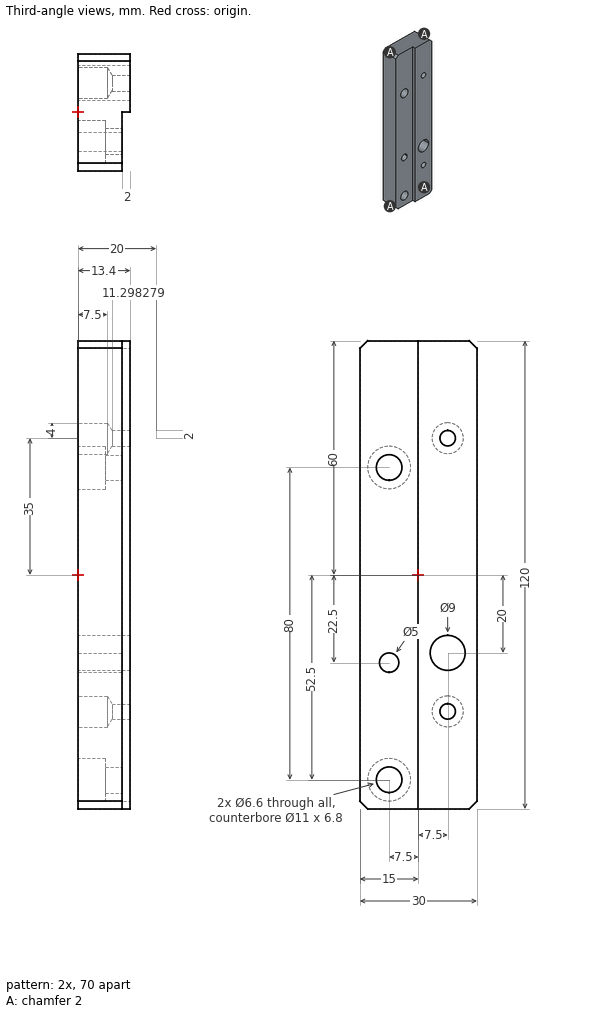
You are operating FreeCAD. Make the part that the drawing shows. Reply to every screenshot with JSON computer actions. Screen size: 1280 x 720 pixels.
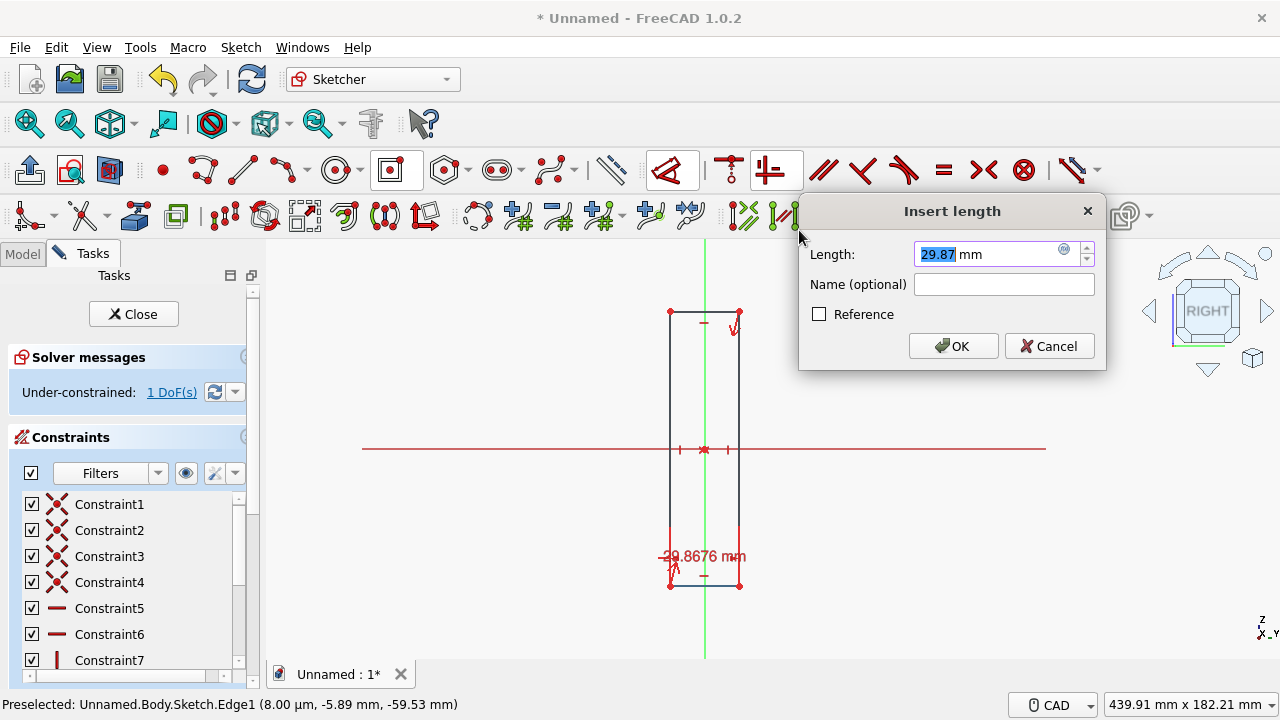
{"action": "type", "text": "30"}
{"action": "key", "text": "Return"}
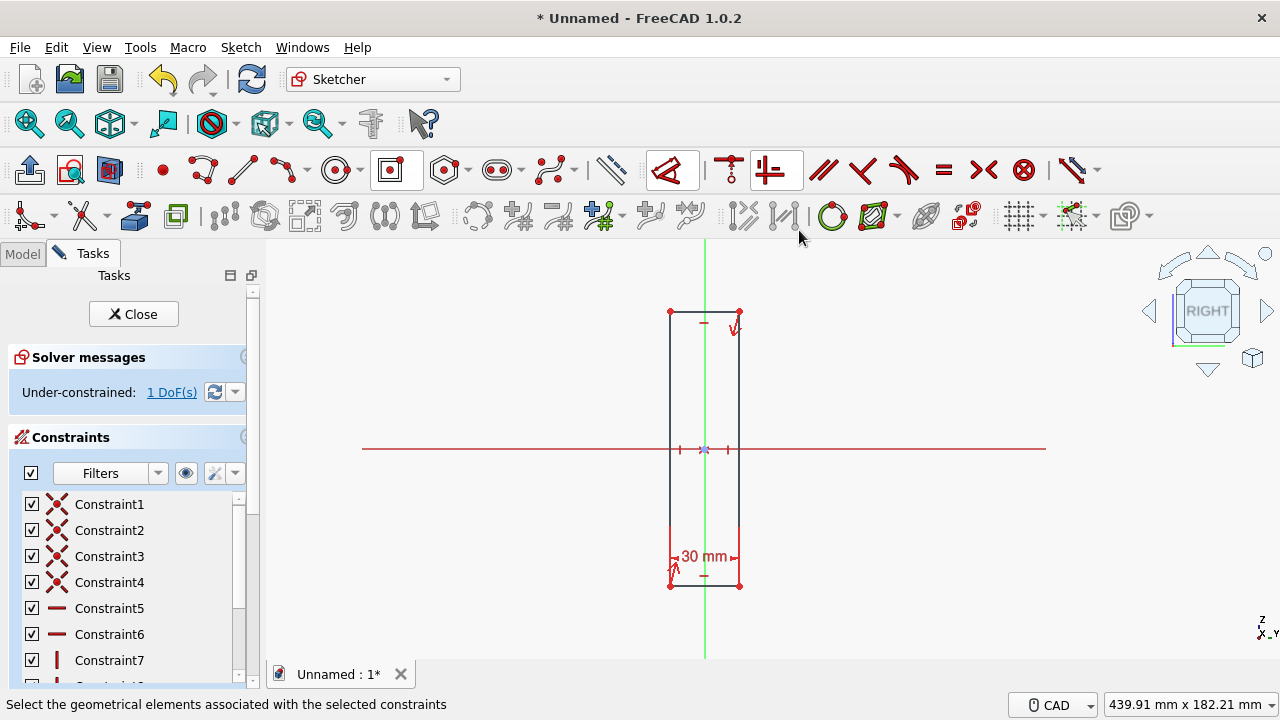
{"action": "left_click", "coordinate": [739, 504]}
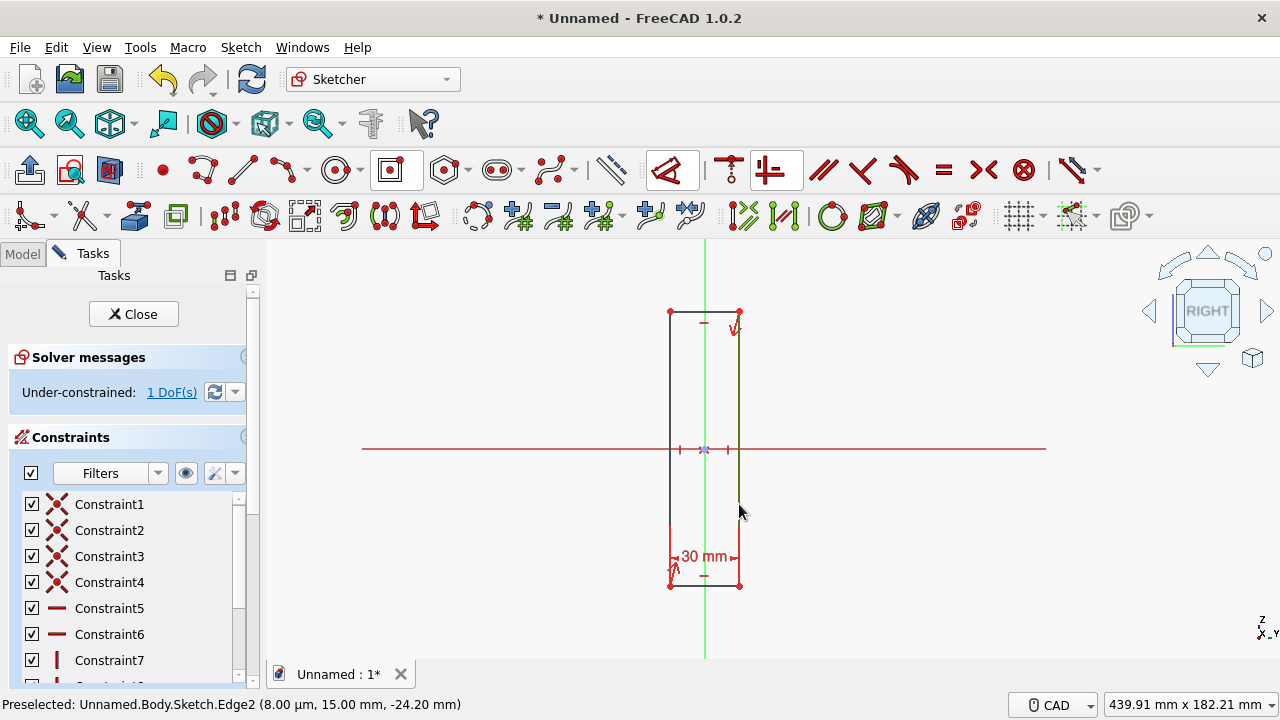
{"action": "key", "text": "i"}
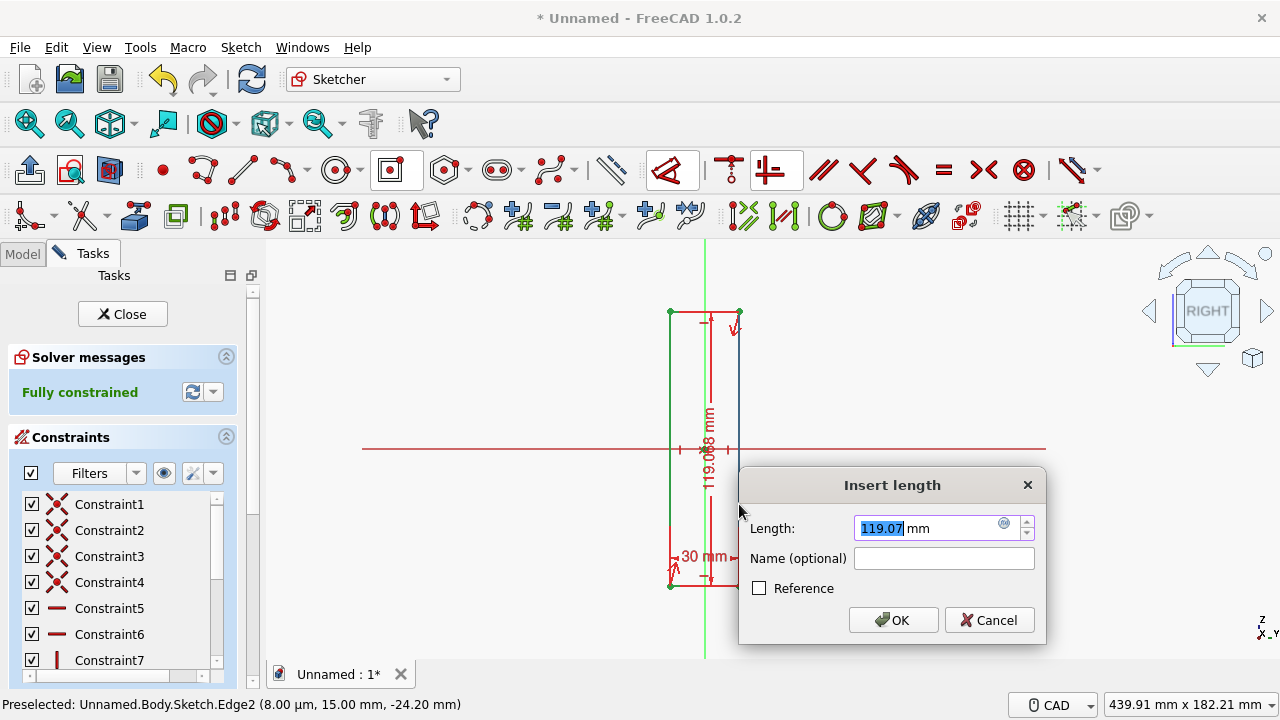
{"action": "type", "text": "120"}
{"action": "key", "text": "Return"}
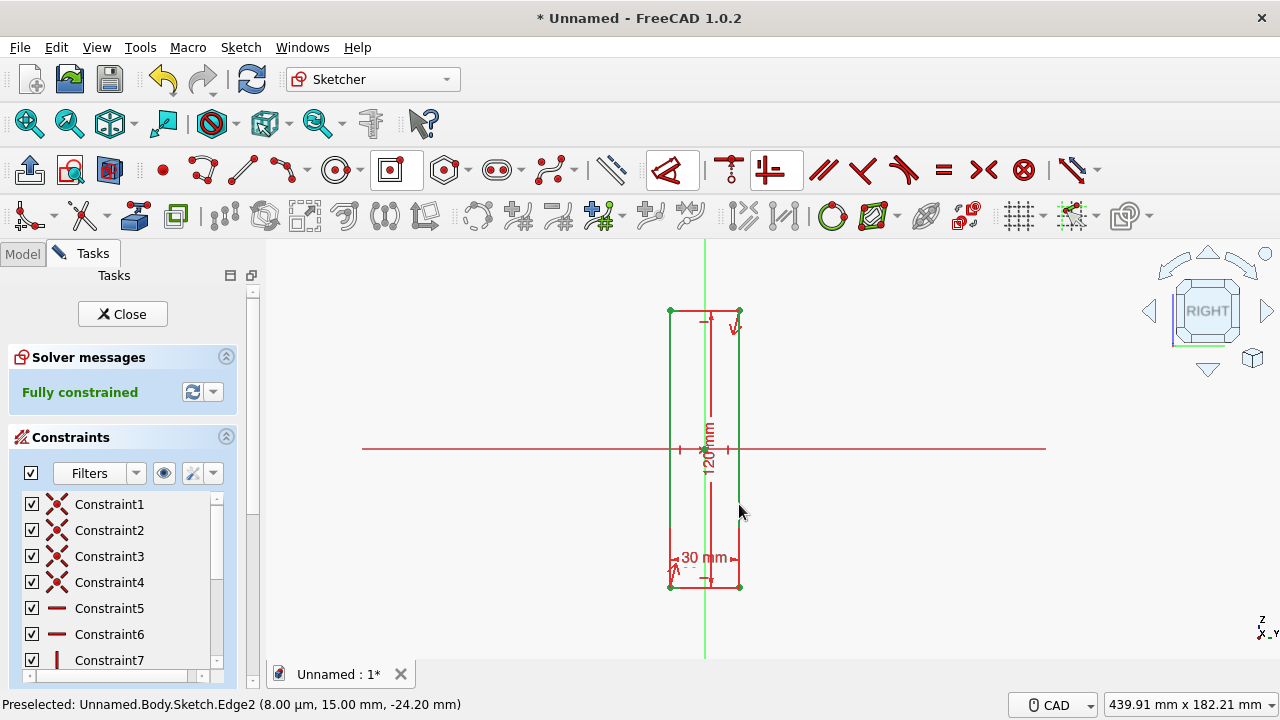
{"action": "left_click", "coordinate": [123, 314]}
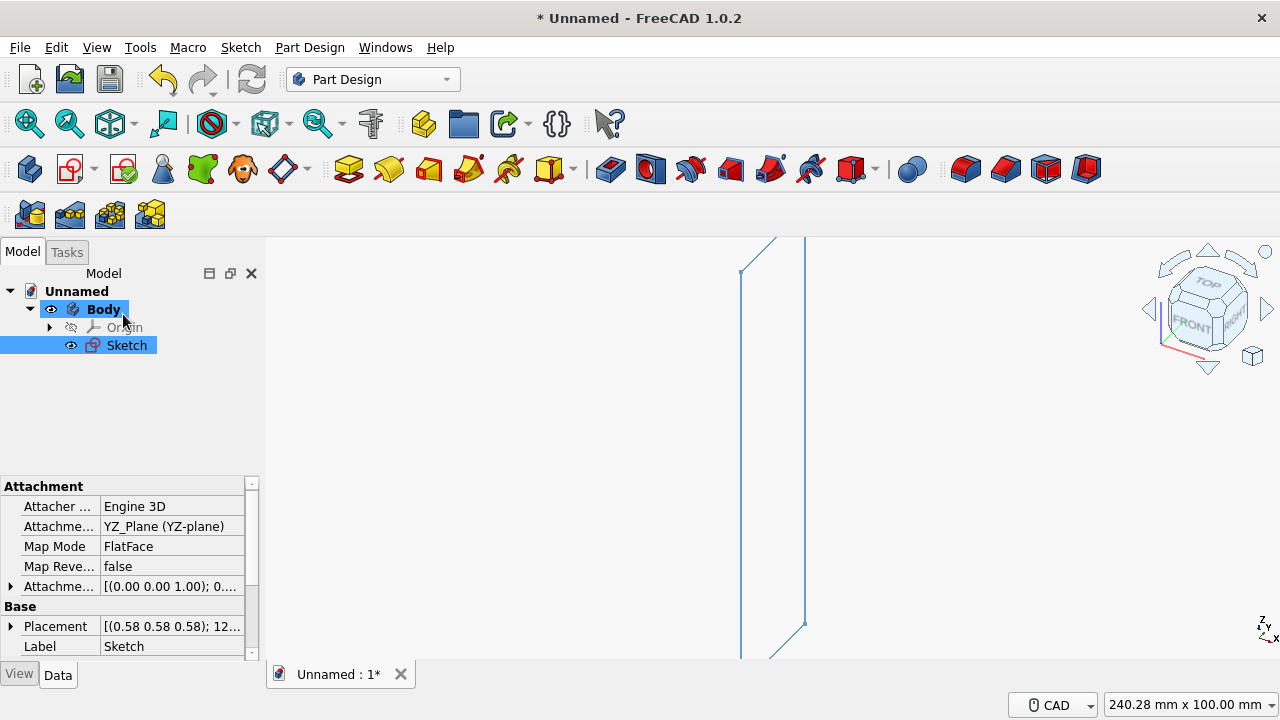
{"action": "left_click", "coordinate": [350, 170]}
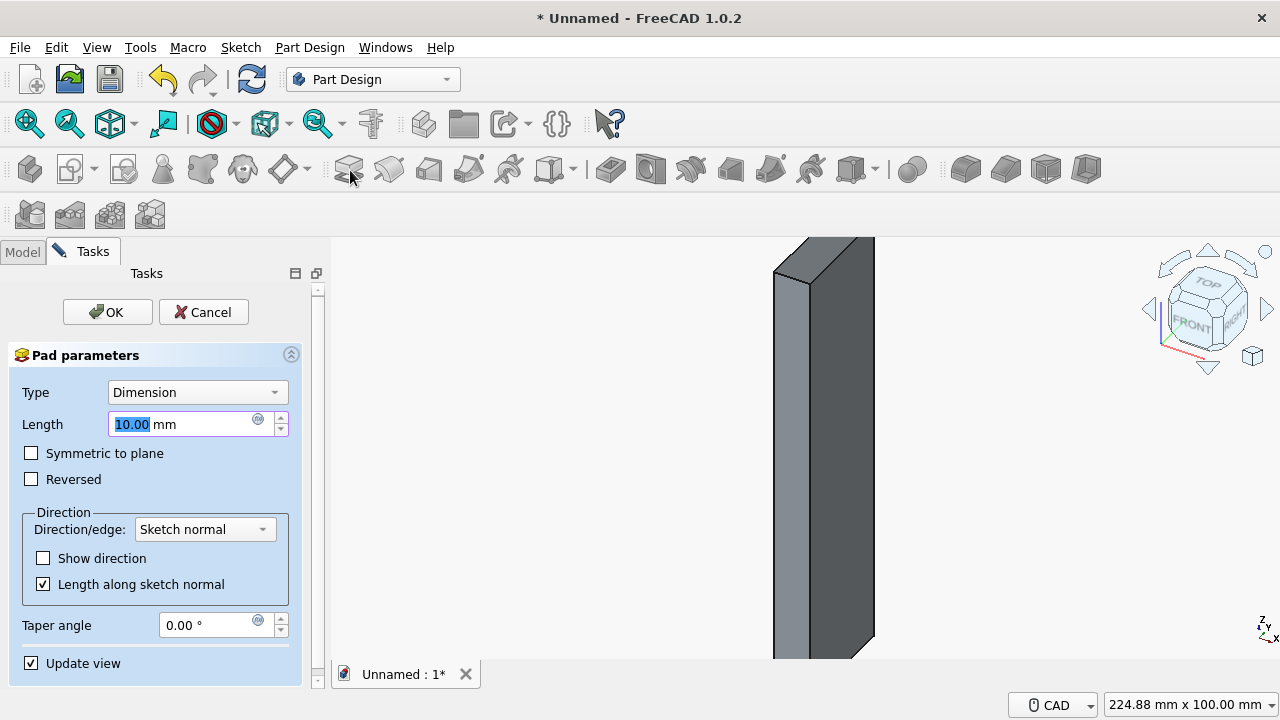
{"action": "type", "text": "13.4"}
{"action": "key", "text": "Tab"}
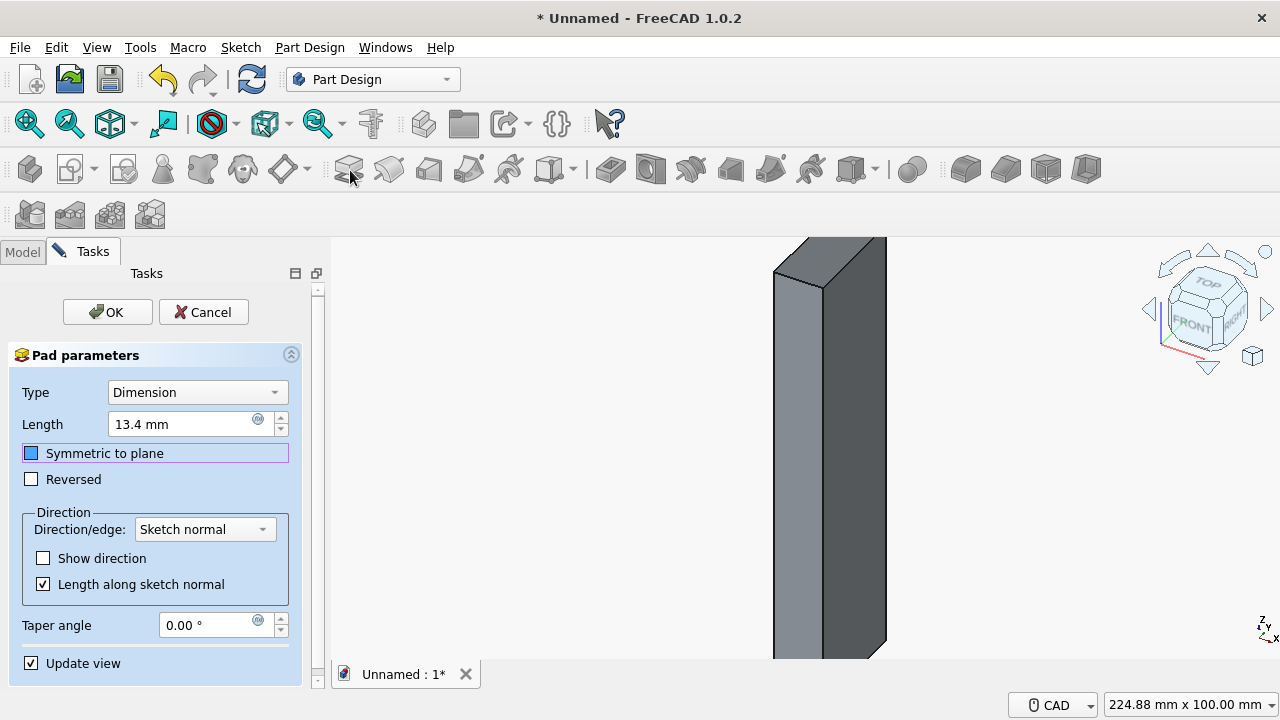
{"action": "left_click", "coordinate": [108, 312]}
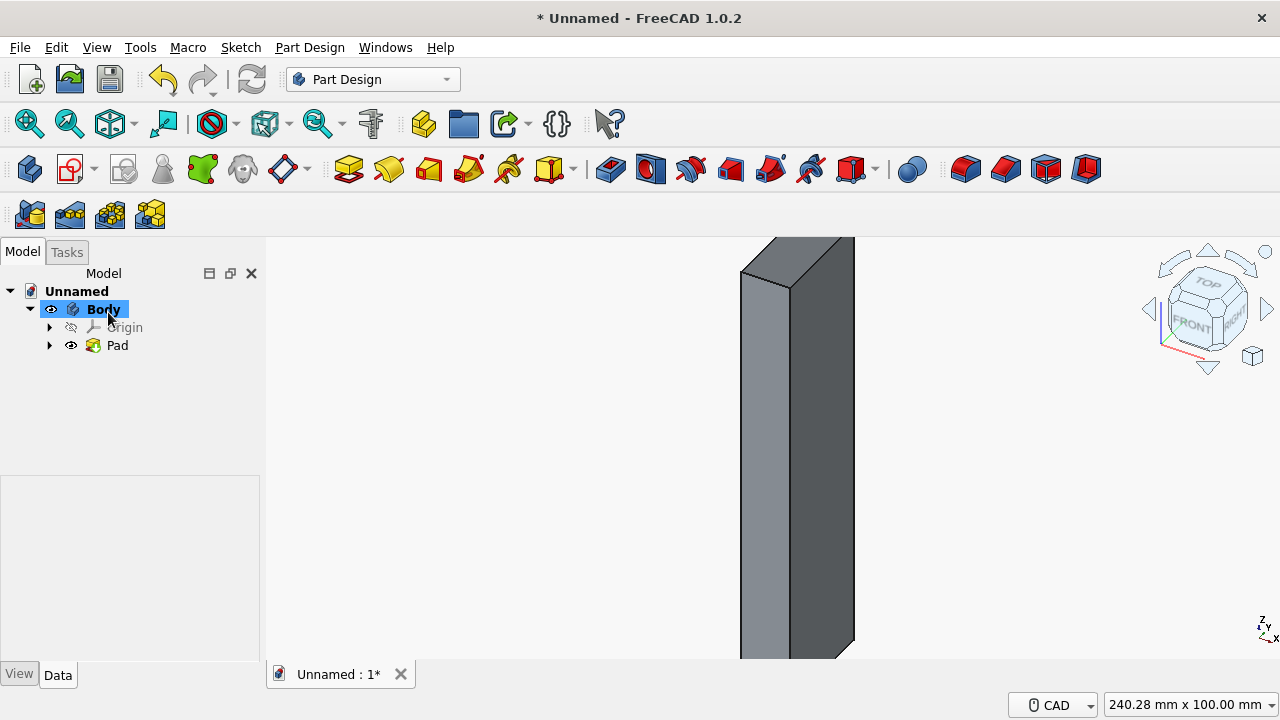
{"action": "left_click", "coordinate": [30, 124]}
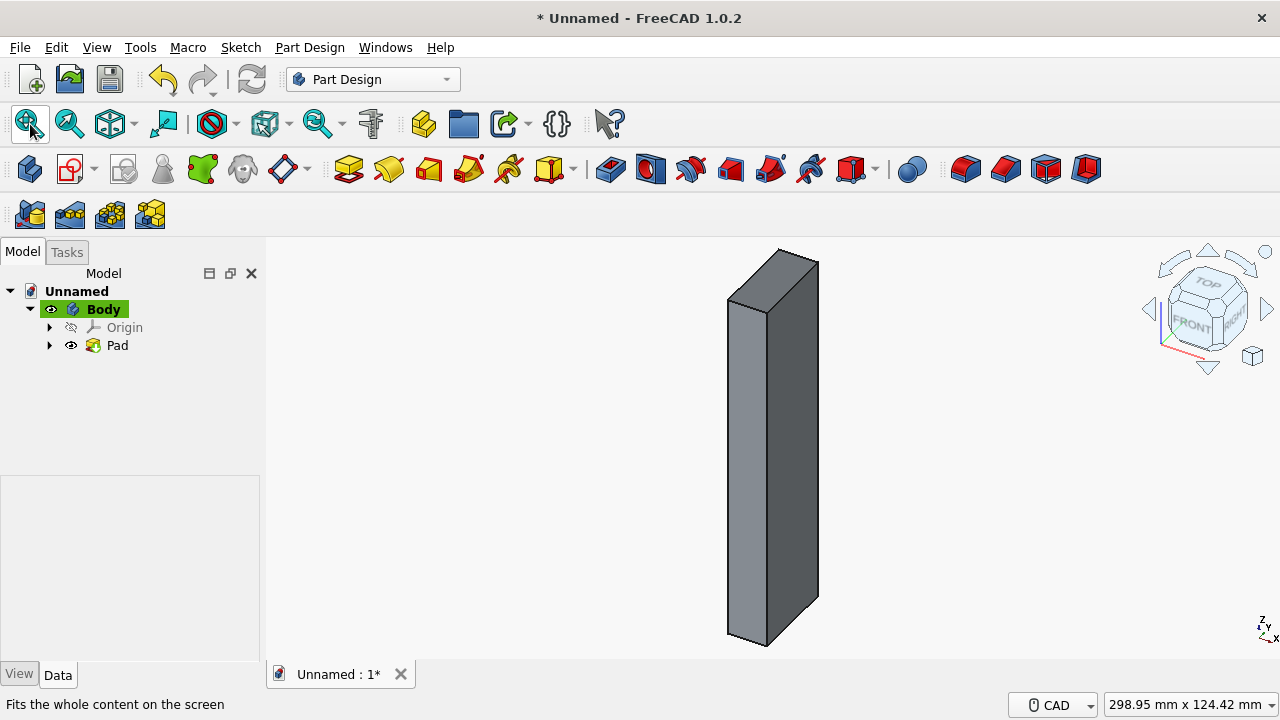
{"action": "left_click", "coordinate": [793, 549]}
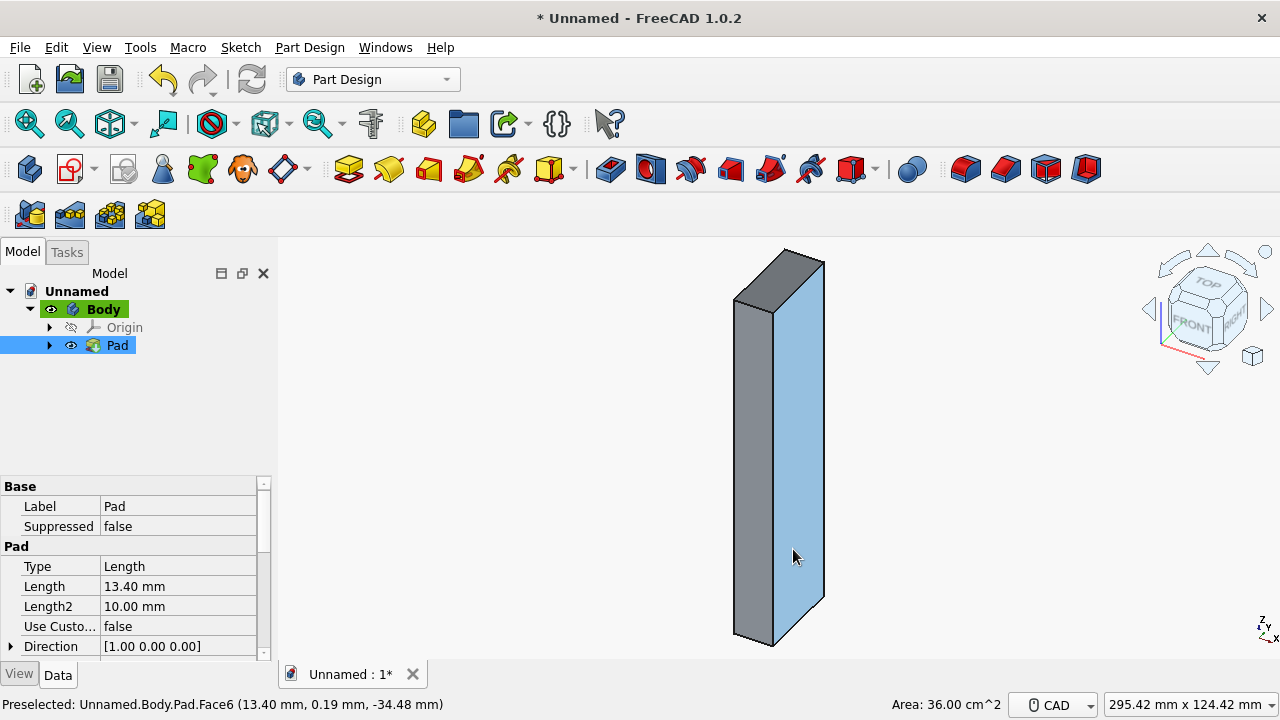
{"action": "left_click", "coordinate": [70, 170]}